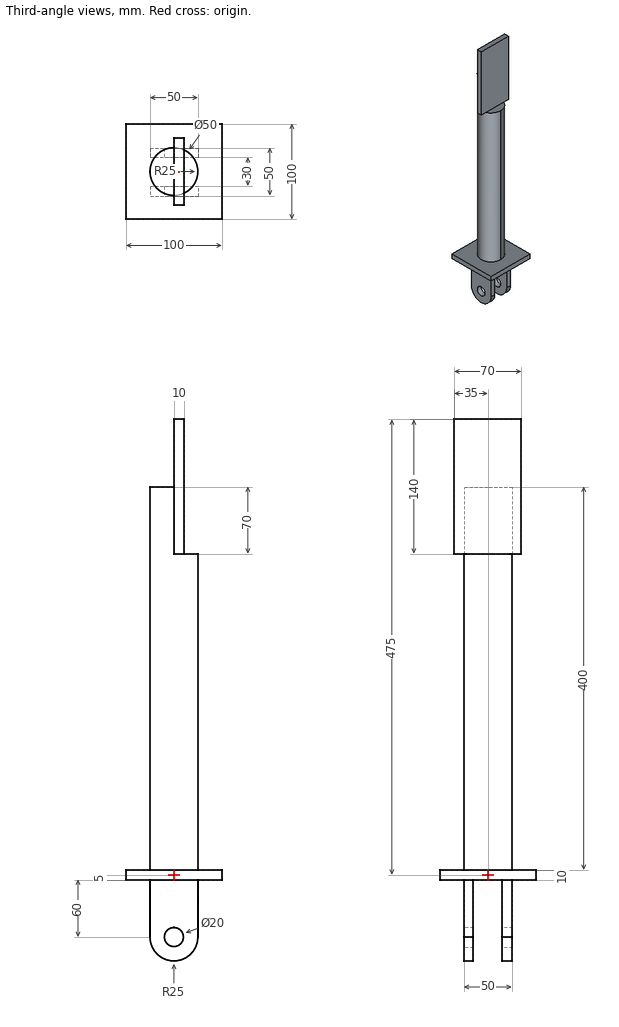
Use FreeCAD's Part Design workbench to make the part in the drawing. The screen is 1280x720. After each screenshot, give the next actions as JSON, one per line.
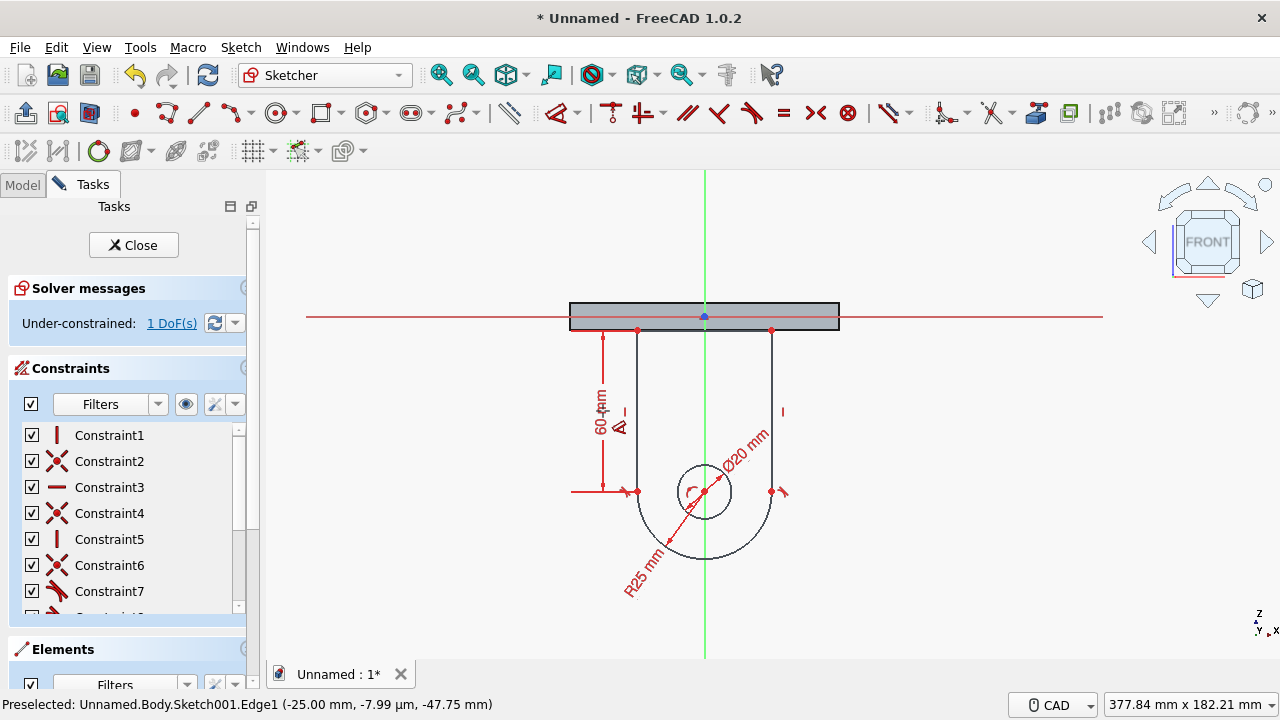
{"action": "scroll", "coordinate": [637, 331], "scroll_direction": "up", "scroll_amount": 6}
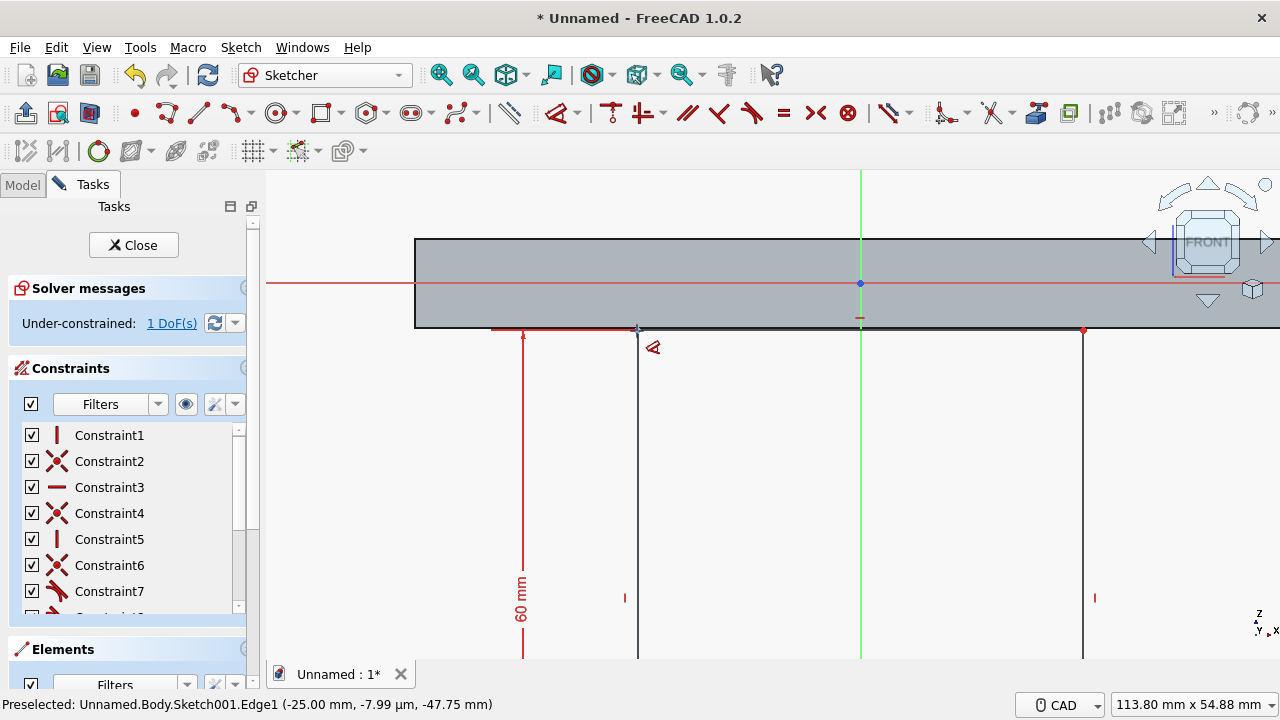
{"action": "left_click", "coordinate": [638, 330]}
{"action": "left_click", "coordinate": [604, 307]}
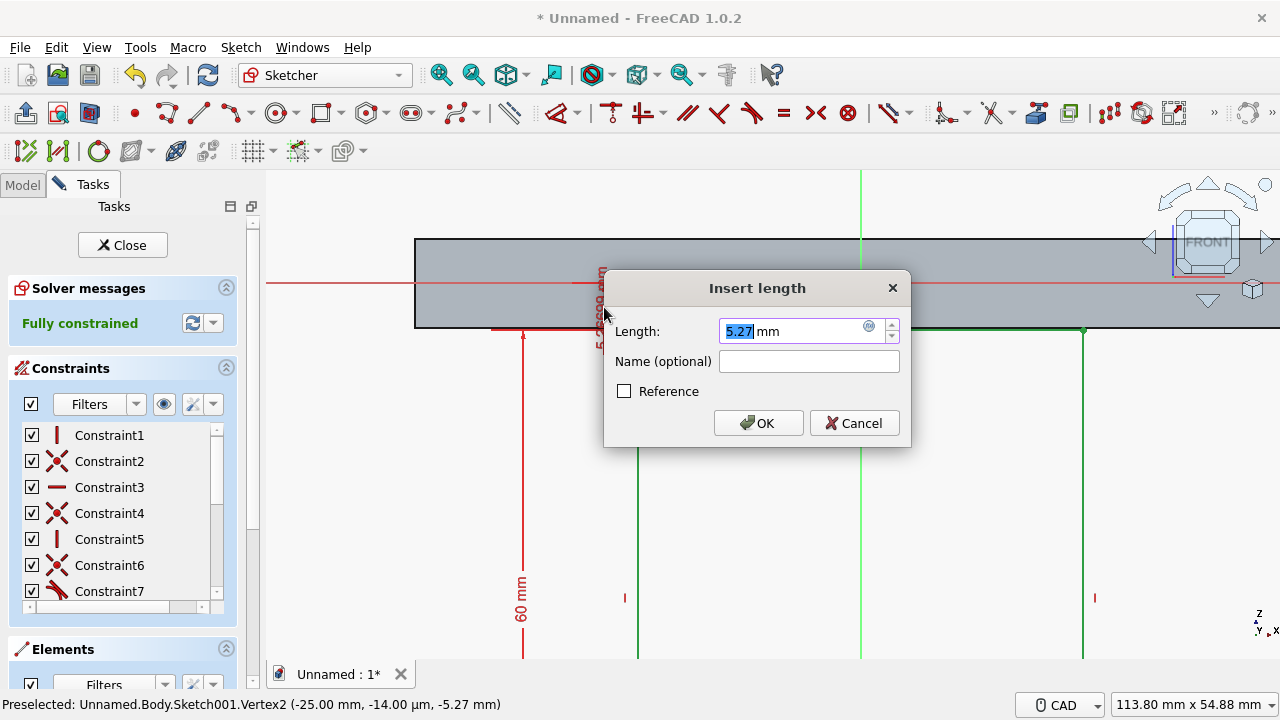
{"action": "type", "text": "5"}
{"action": "key", "text": "Return"}
{"action": "key", "text": "Escape"}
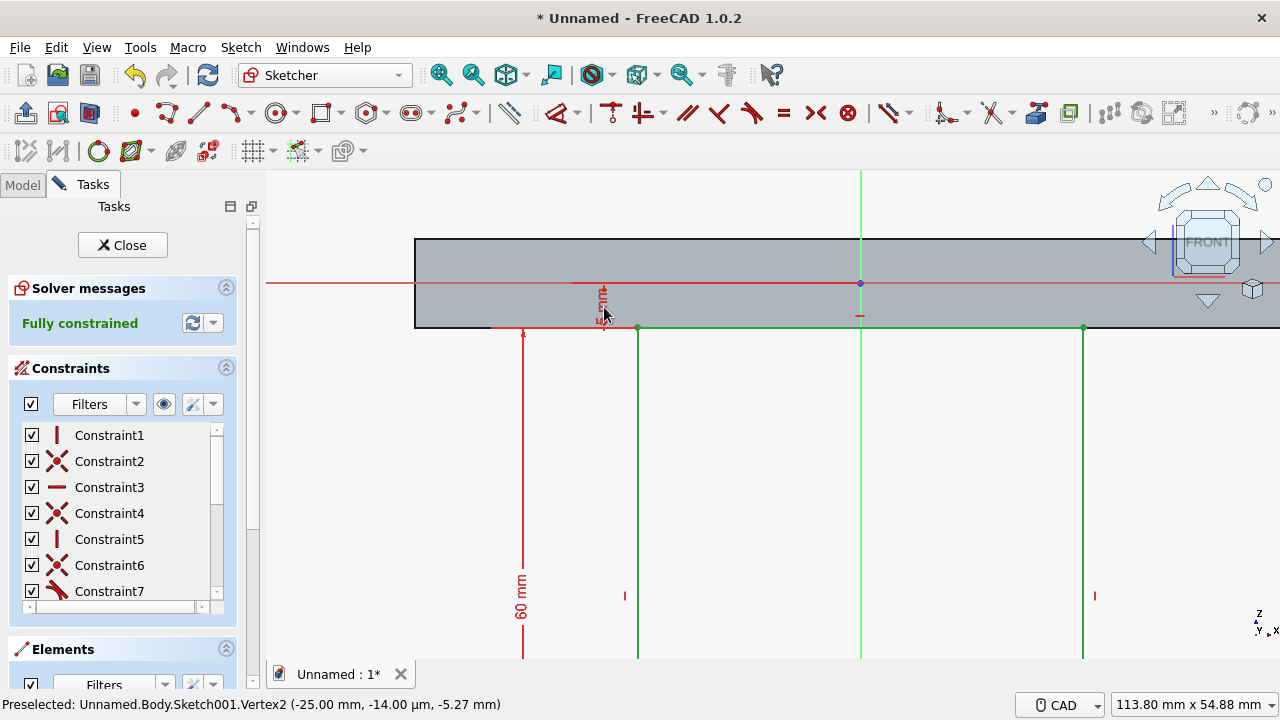
{"action": "left_click", "coordinate": [123, 245]}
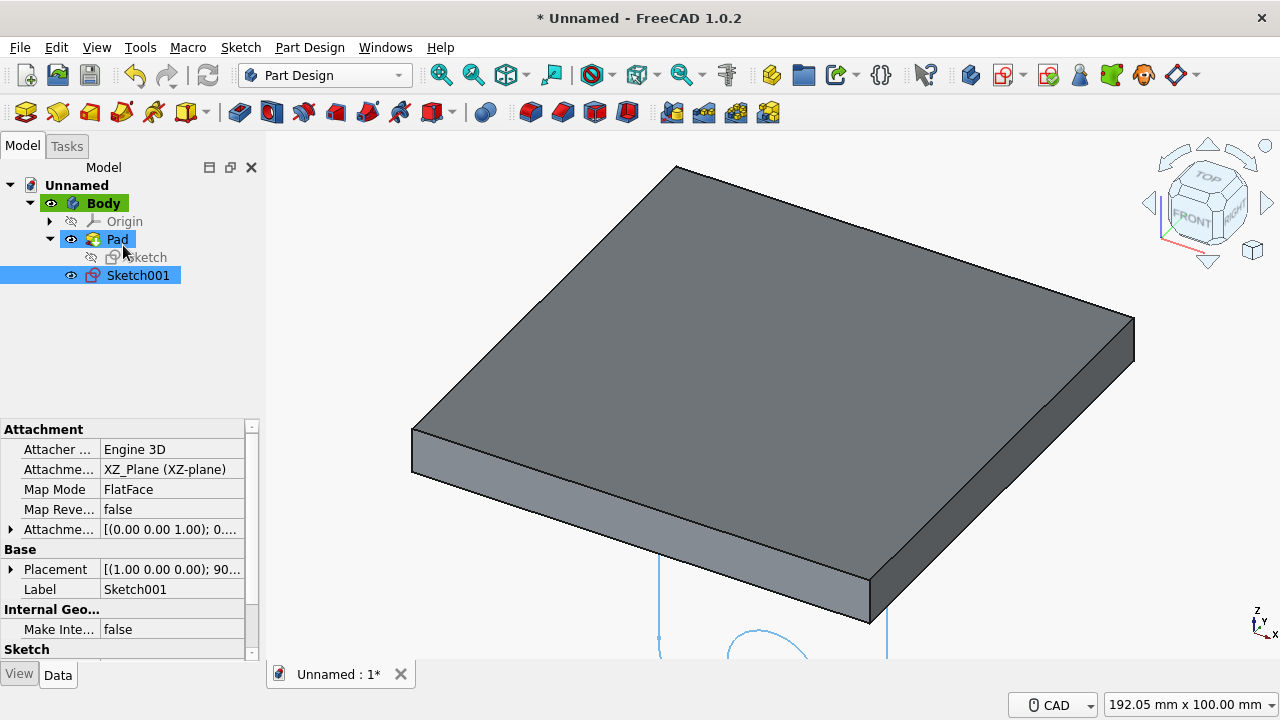
{"action": "left_click", "coordinate": [26, 112]}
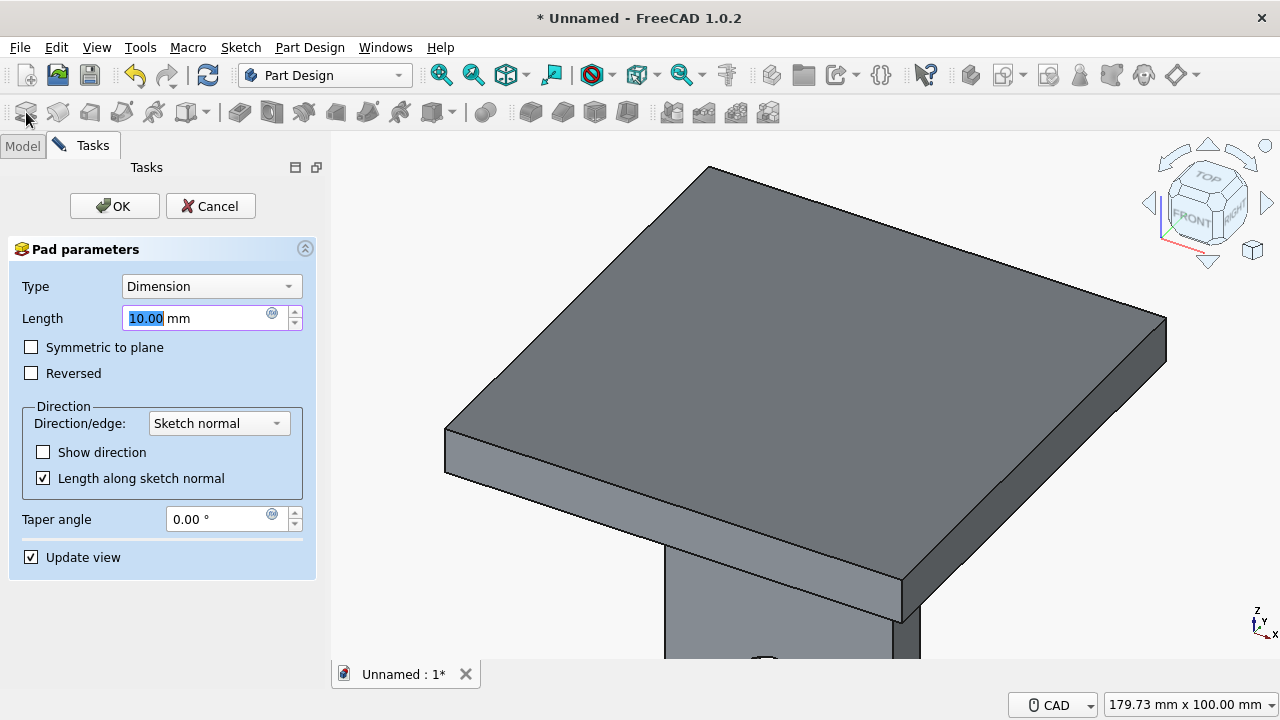
{"action": "type", "text": "50"}
{"action": "key", "text": "Tab"}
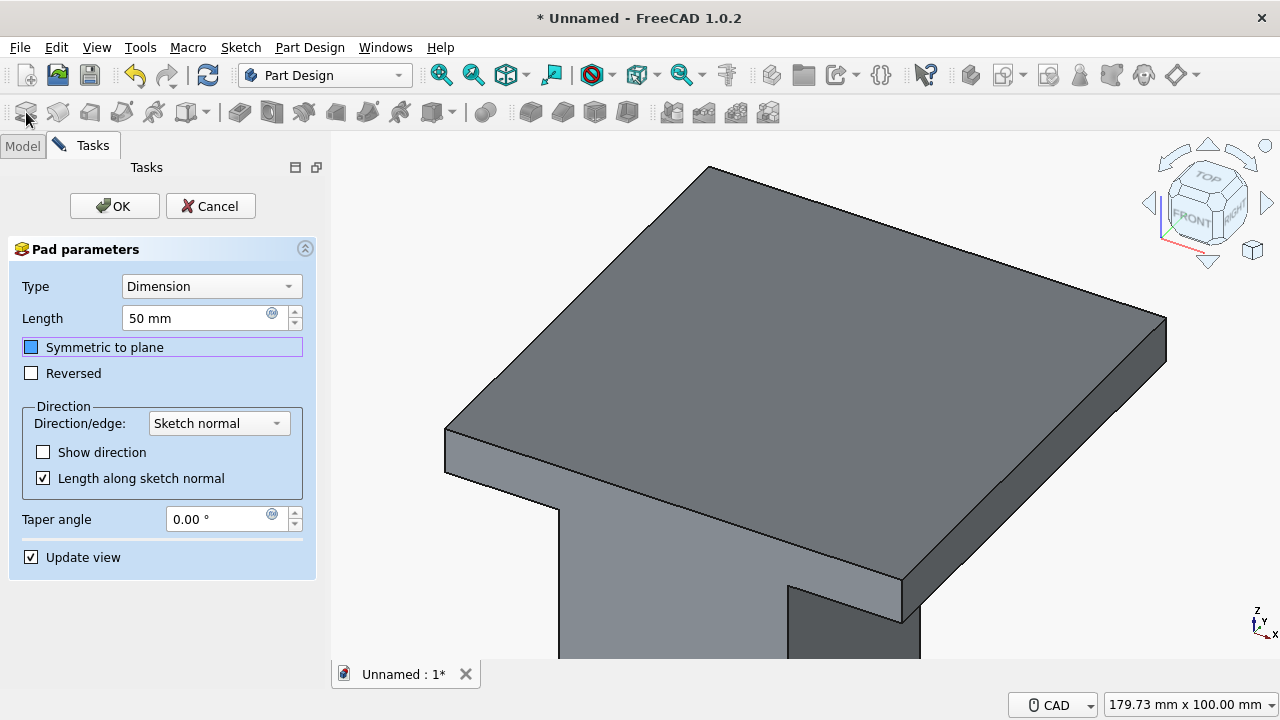
{"action": "left_click", "coordinate": [30, 347]}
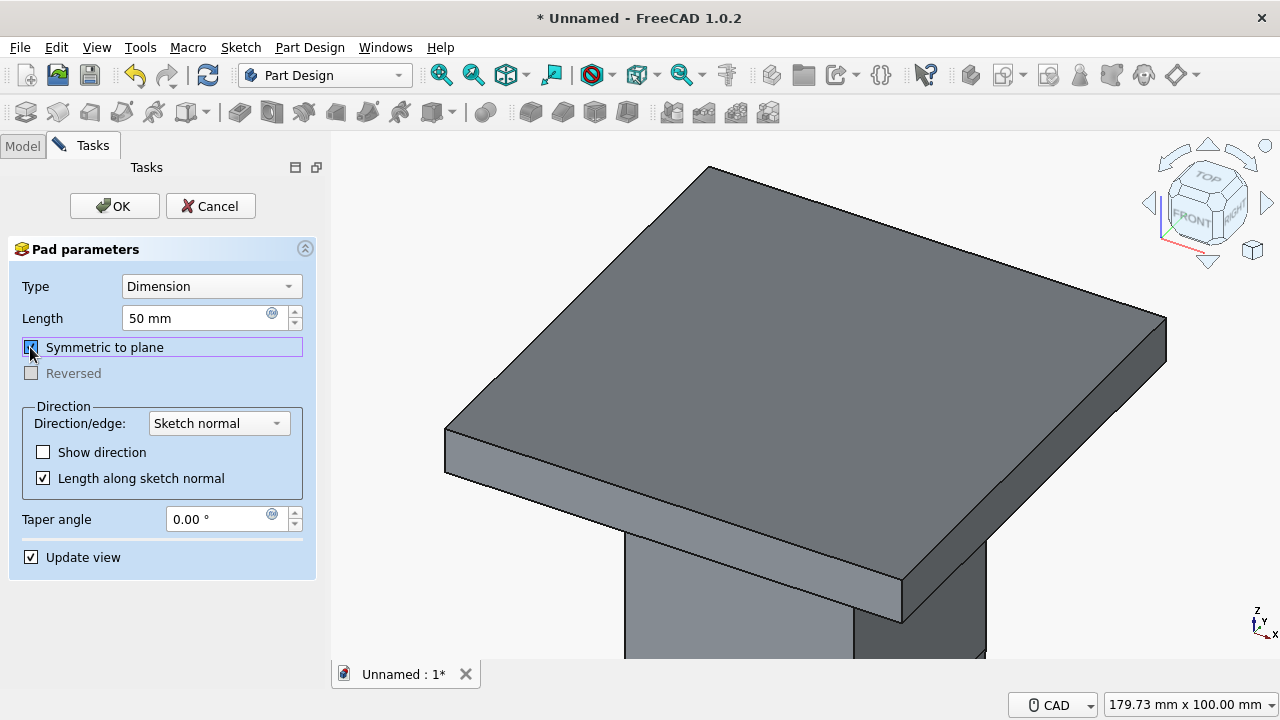
{"action": "left_click", "coordinate": [115, 206]}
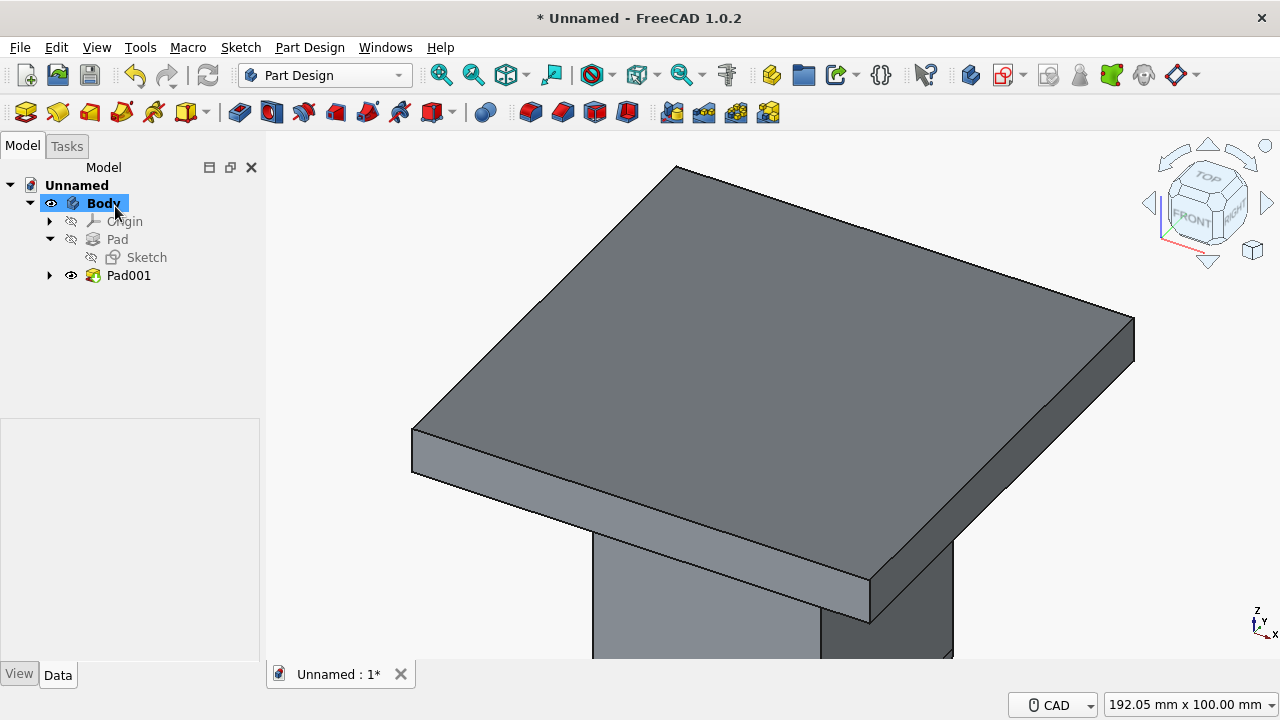
{"action": "key", "text": "v f"}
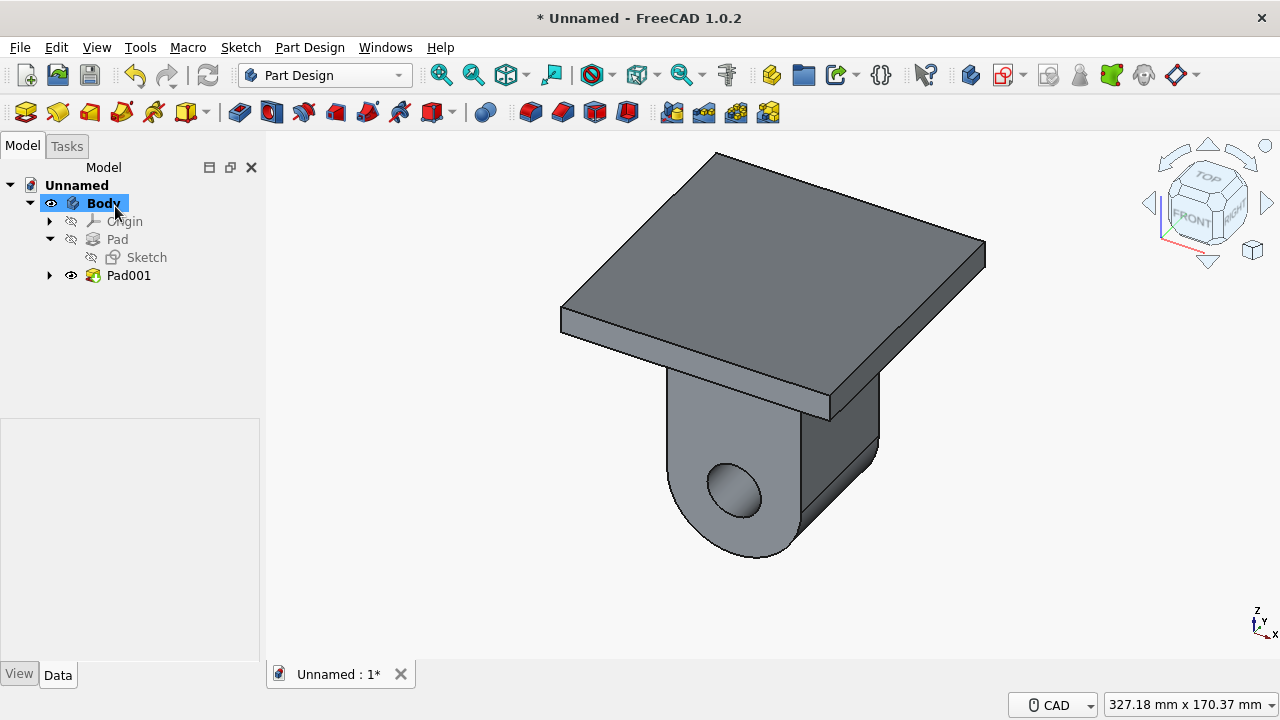
{"action": "key", "text": "5"}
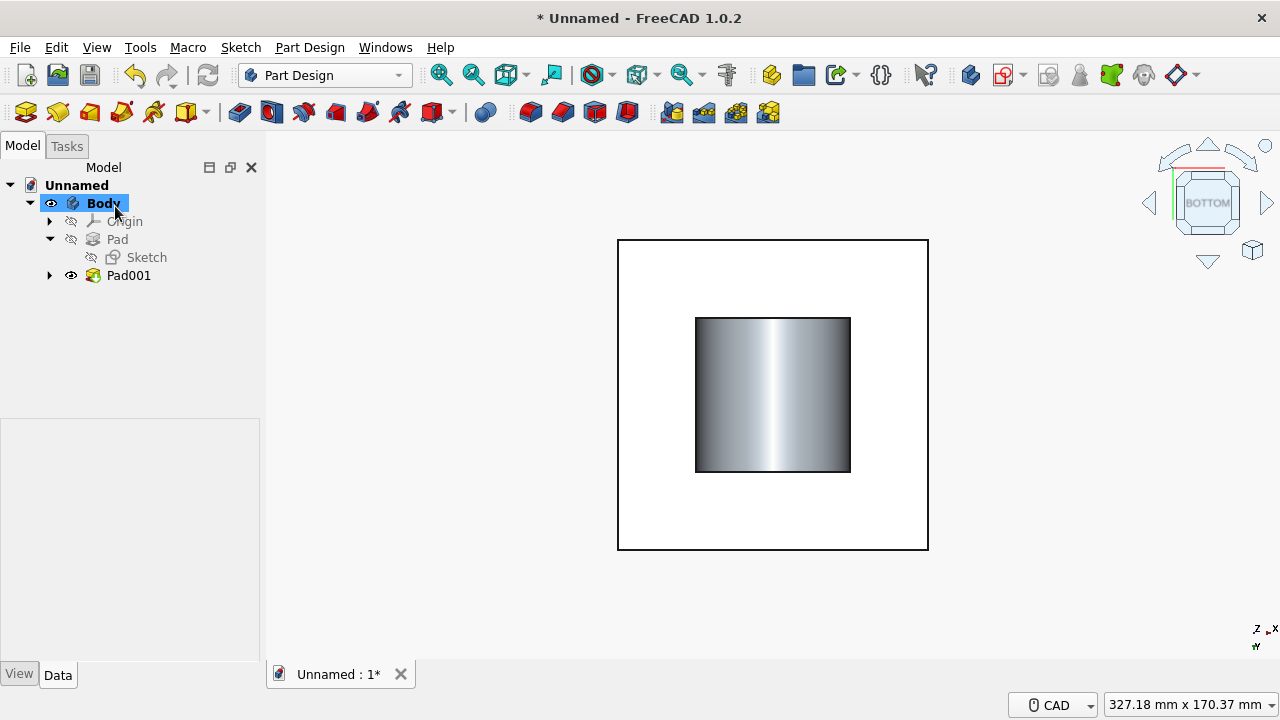
{"action": "left_click", "coordinate": [862, 261]}